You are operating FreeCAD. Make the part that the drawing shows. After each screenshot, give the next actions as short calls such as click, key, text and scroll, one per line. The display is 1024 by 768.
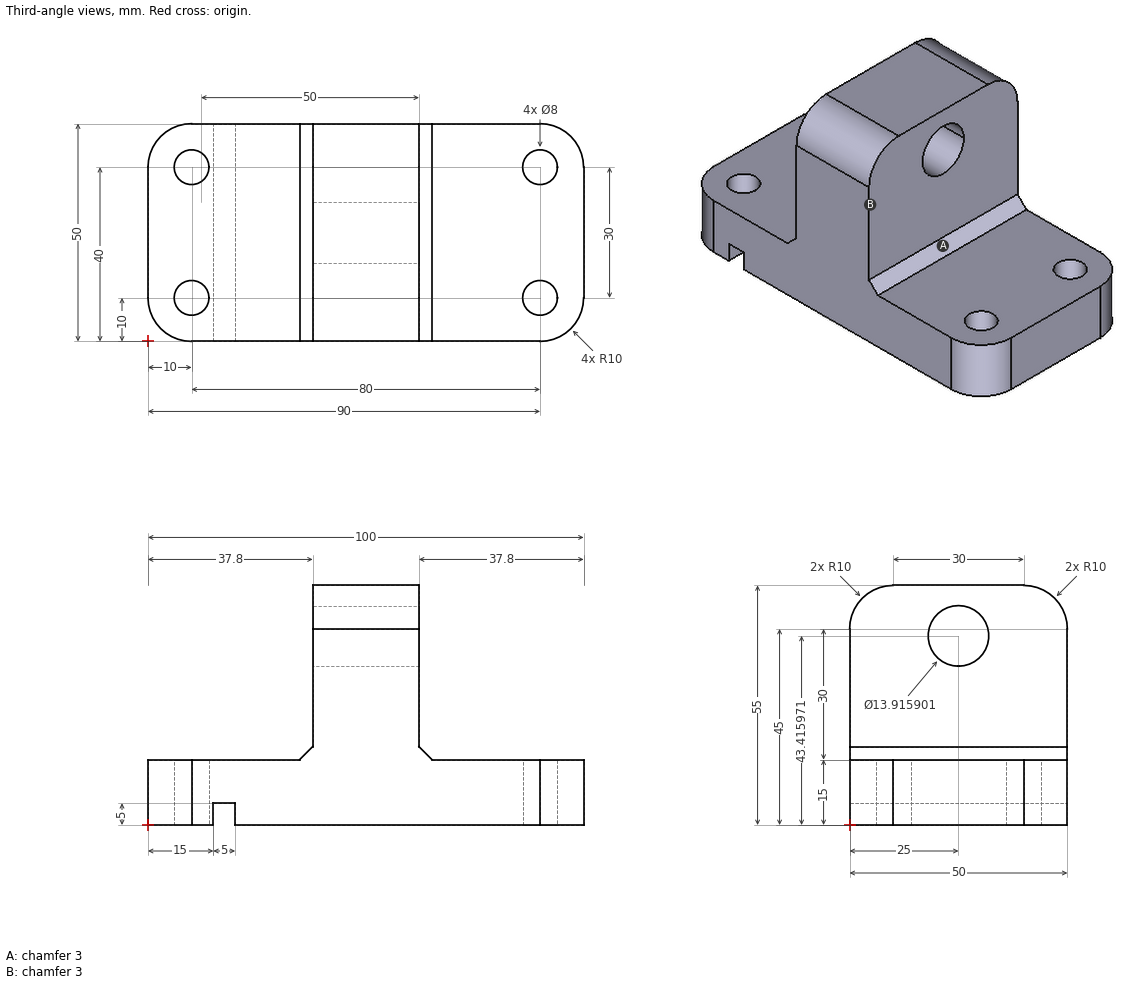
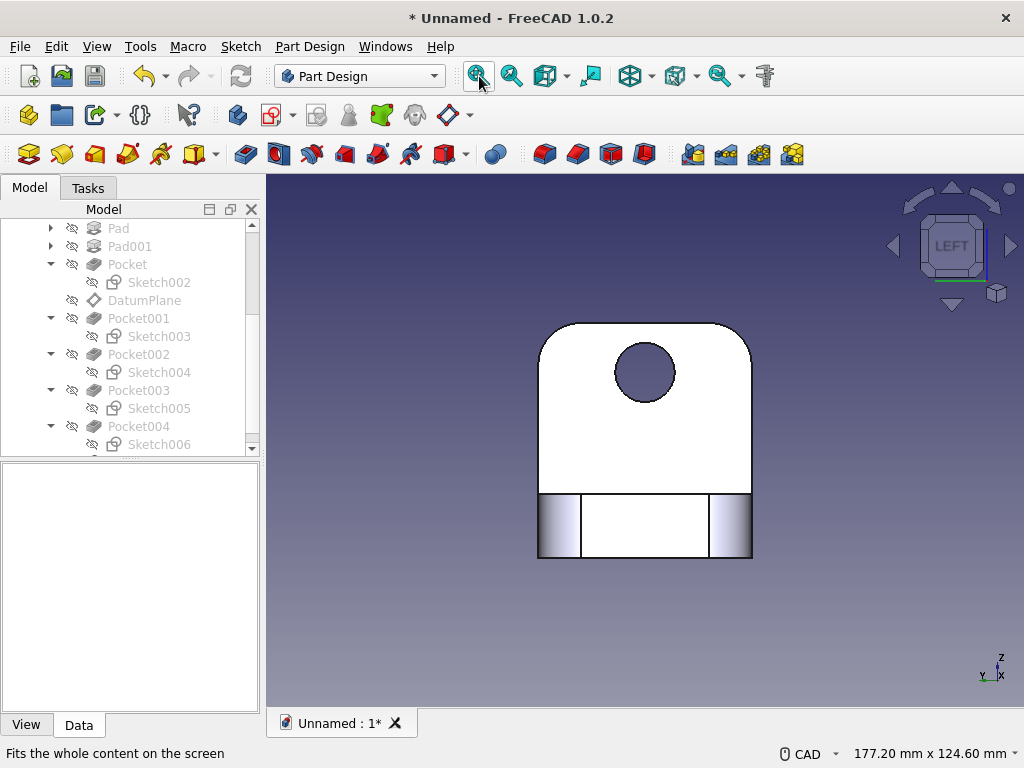
key(0)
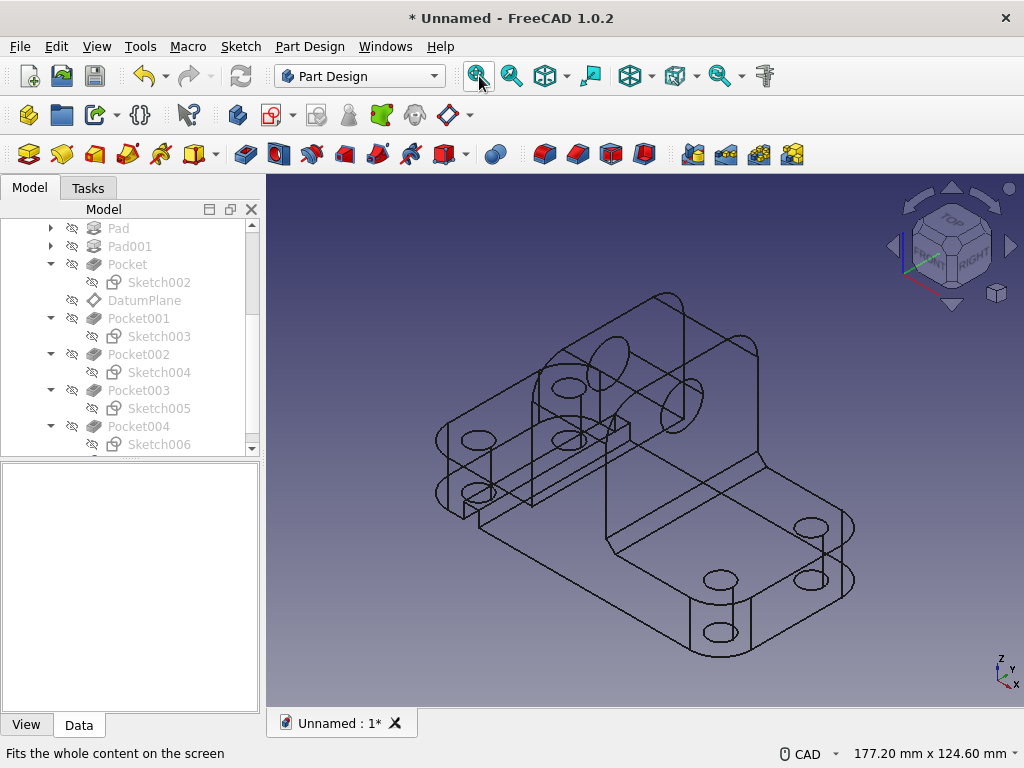
click(623, 453)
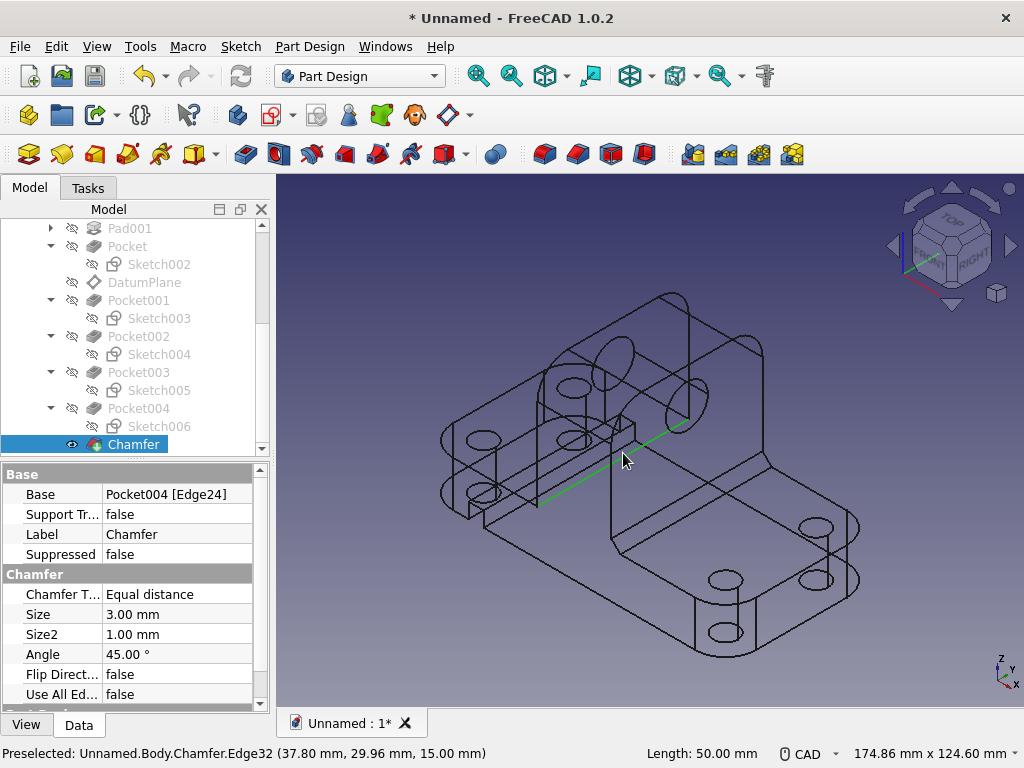
key(v)
key(1)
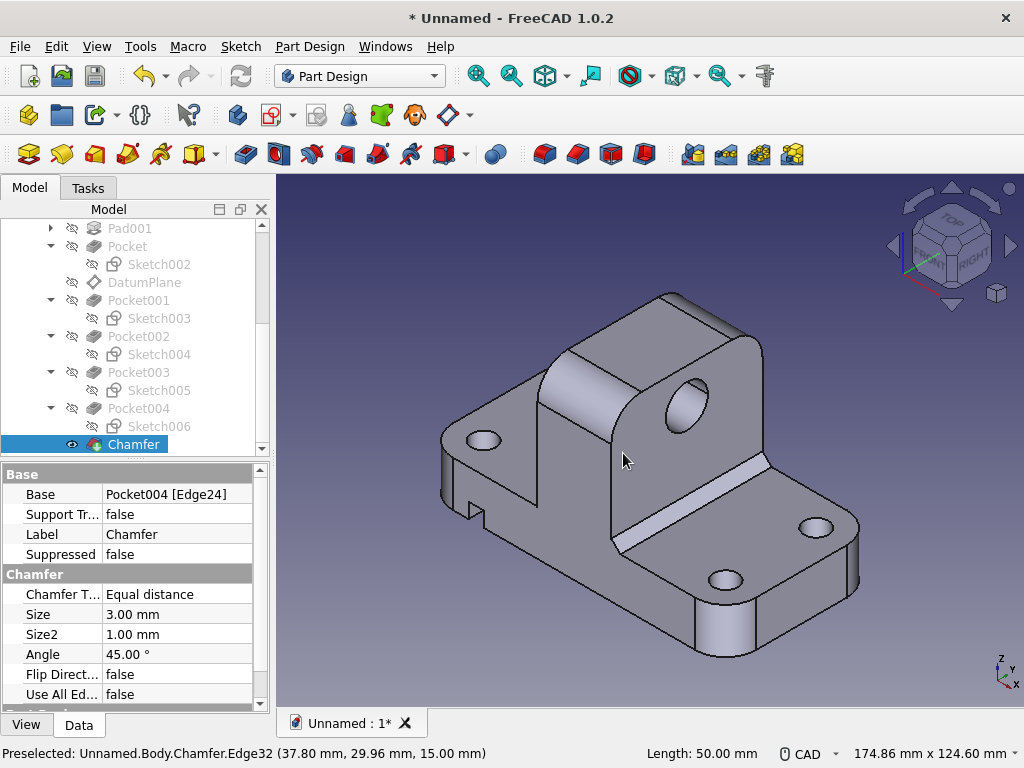
click(578, 154)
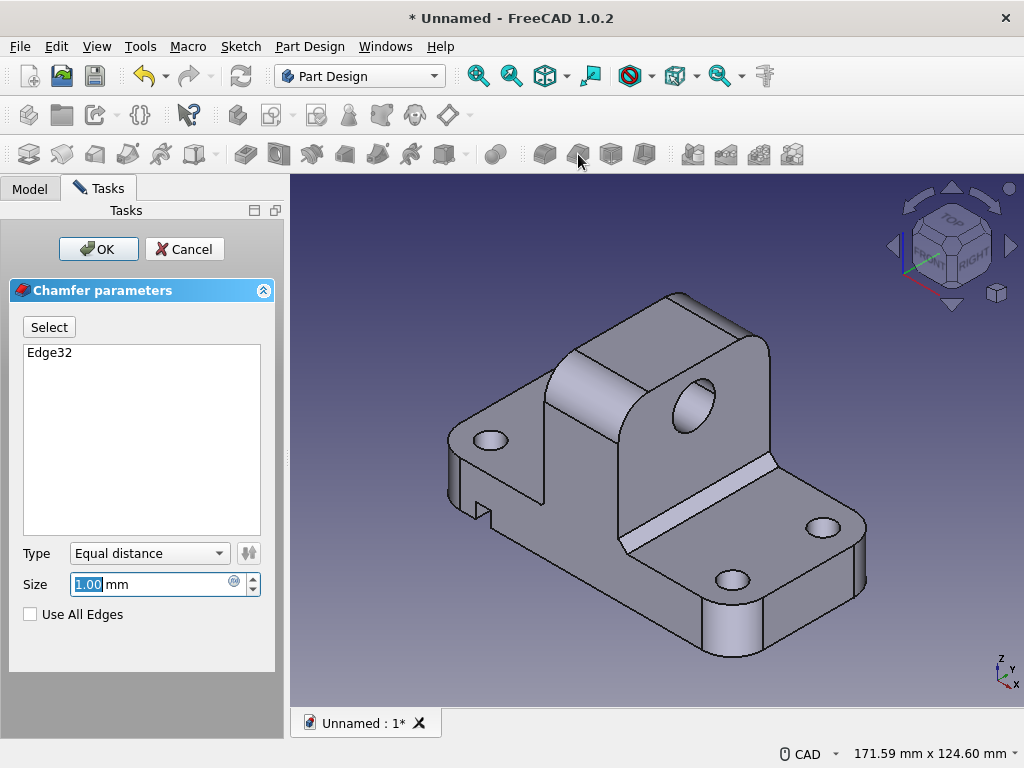
text(3)
key(Tab)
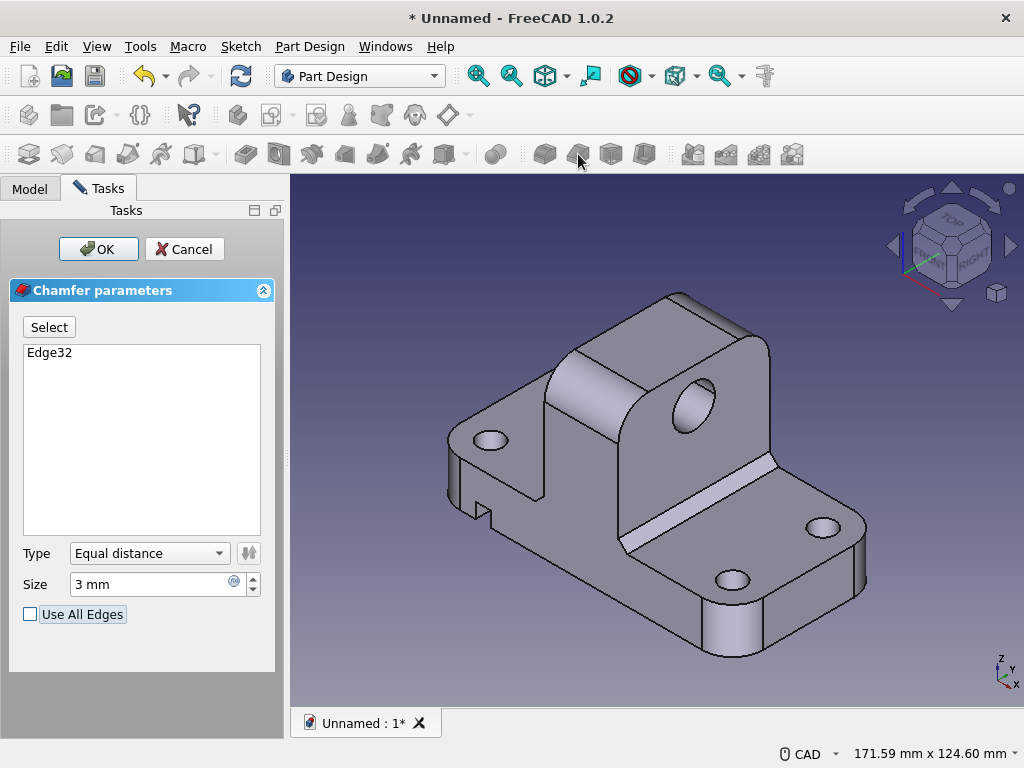
click(99, 249)